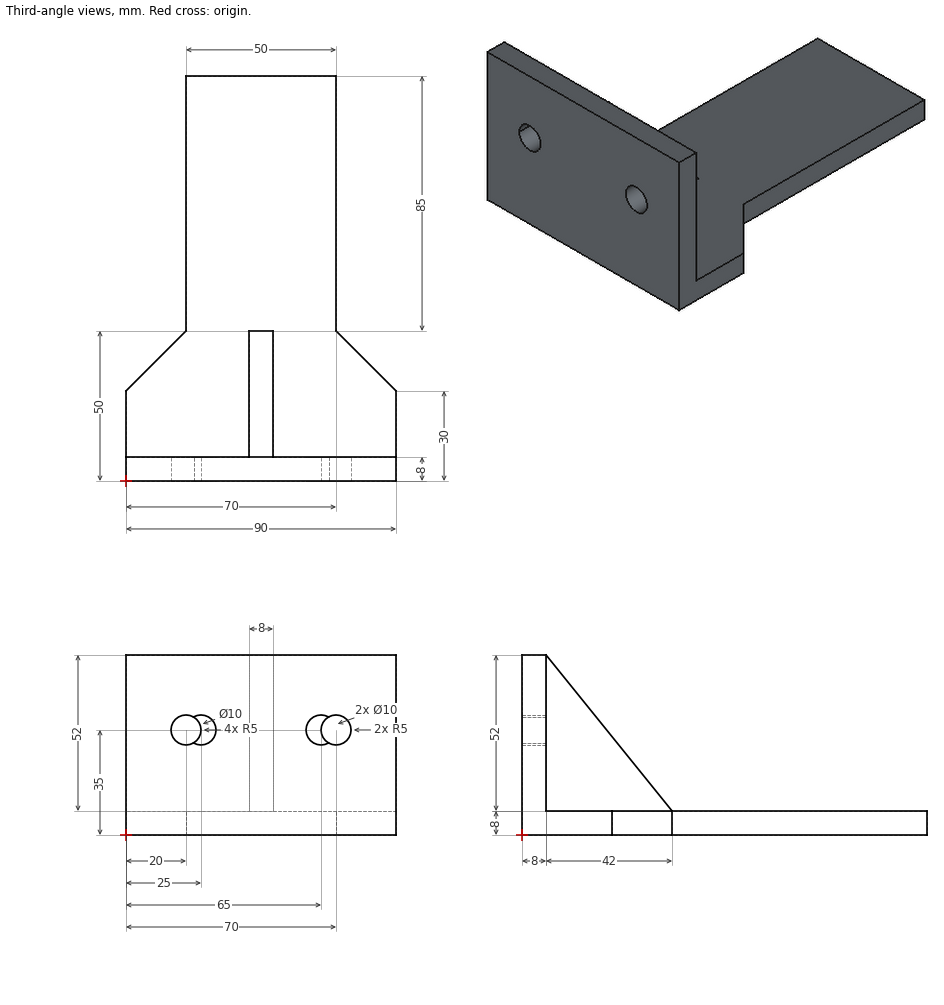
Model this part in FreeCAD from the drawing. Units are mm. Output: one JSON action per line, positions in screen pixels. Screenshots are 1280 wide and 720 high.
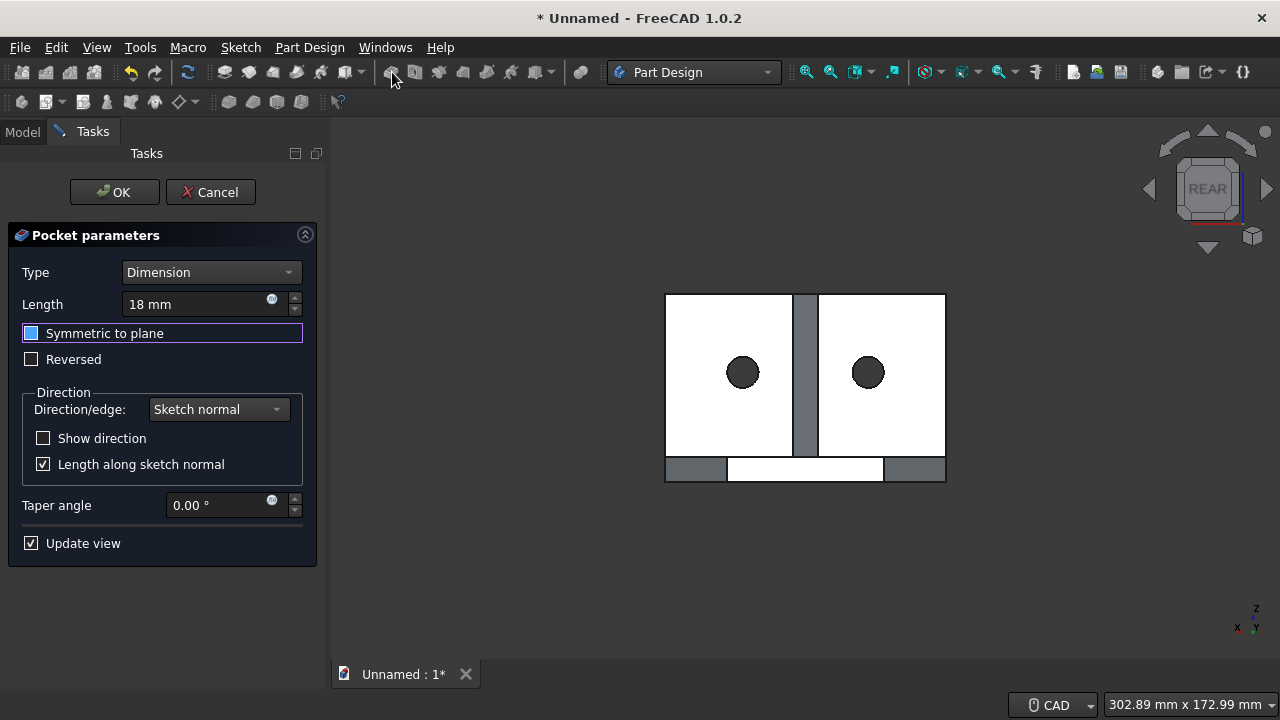
{"action": "left_click", "coordinate": [115, 192]}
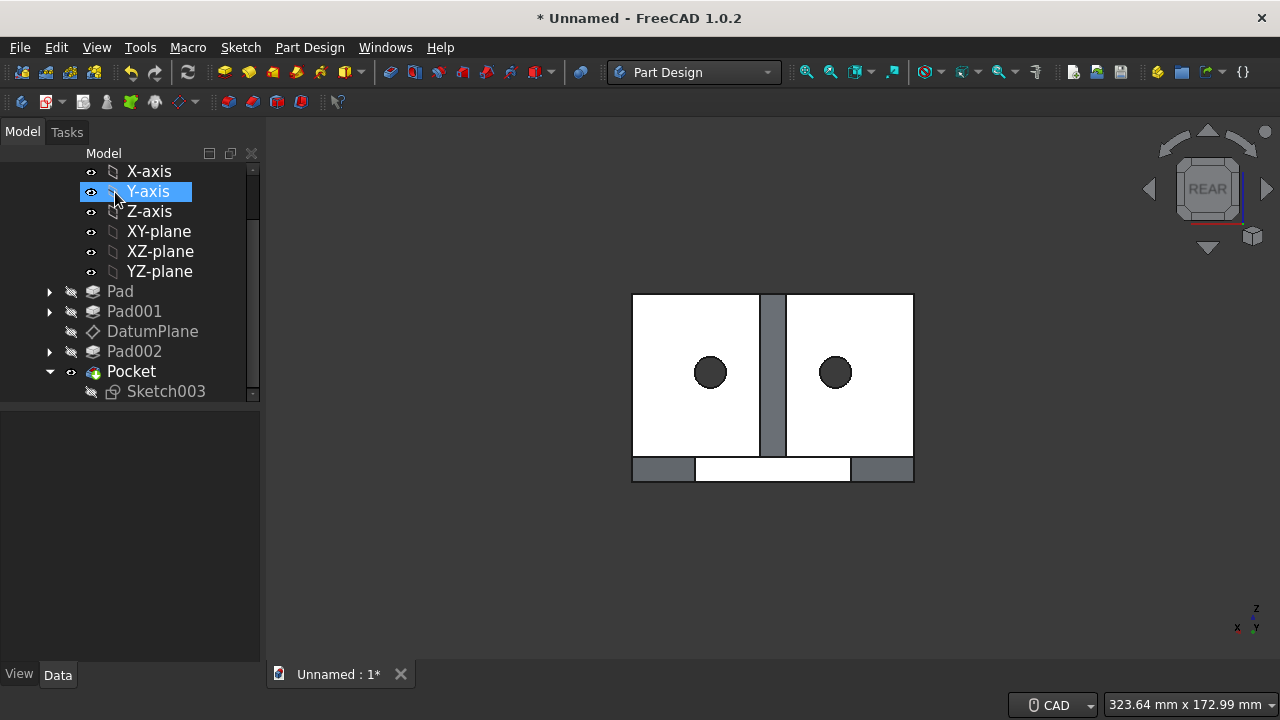
{"action": "left_click", "coordinate": [808, 72]}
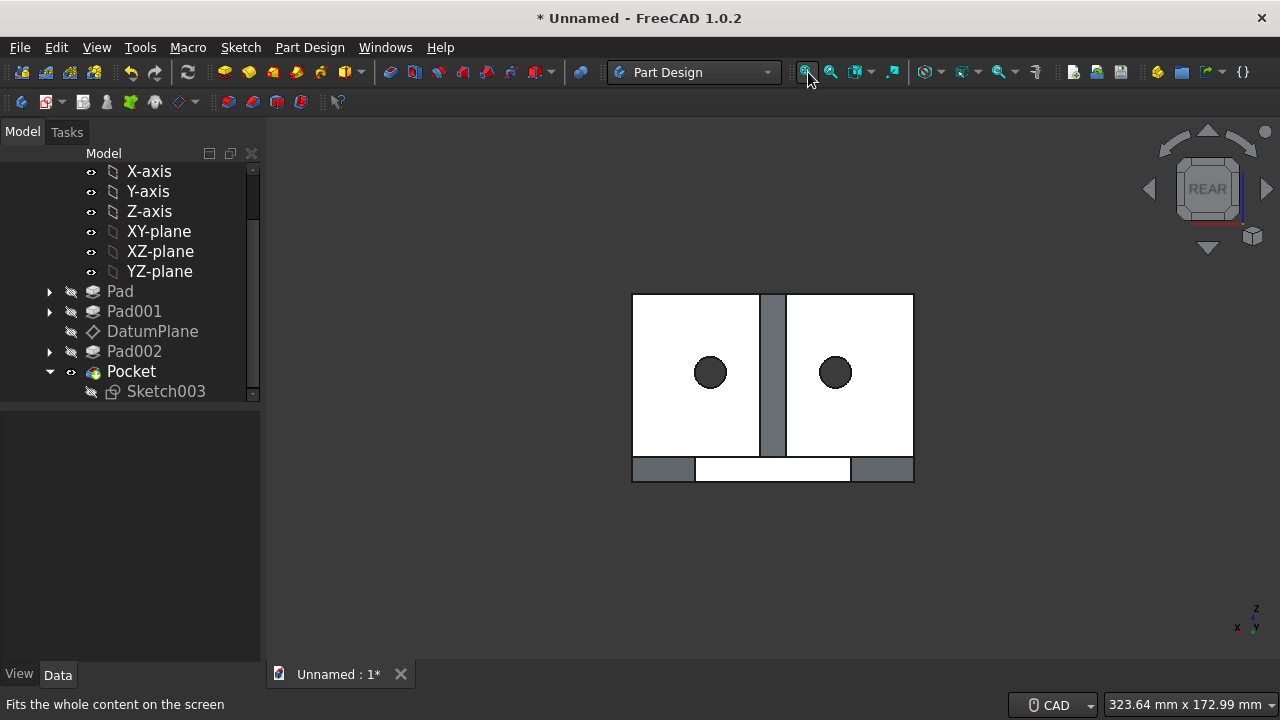
{"action": "left_click", "coordinate": [850, 421]}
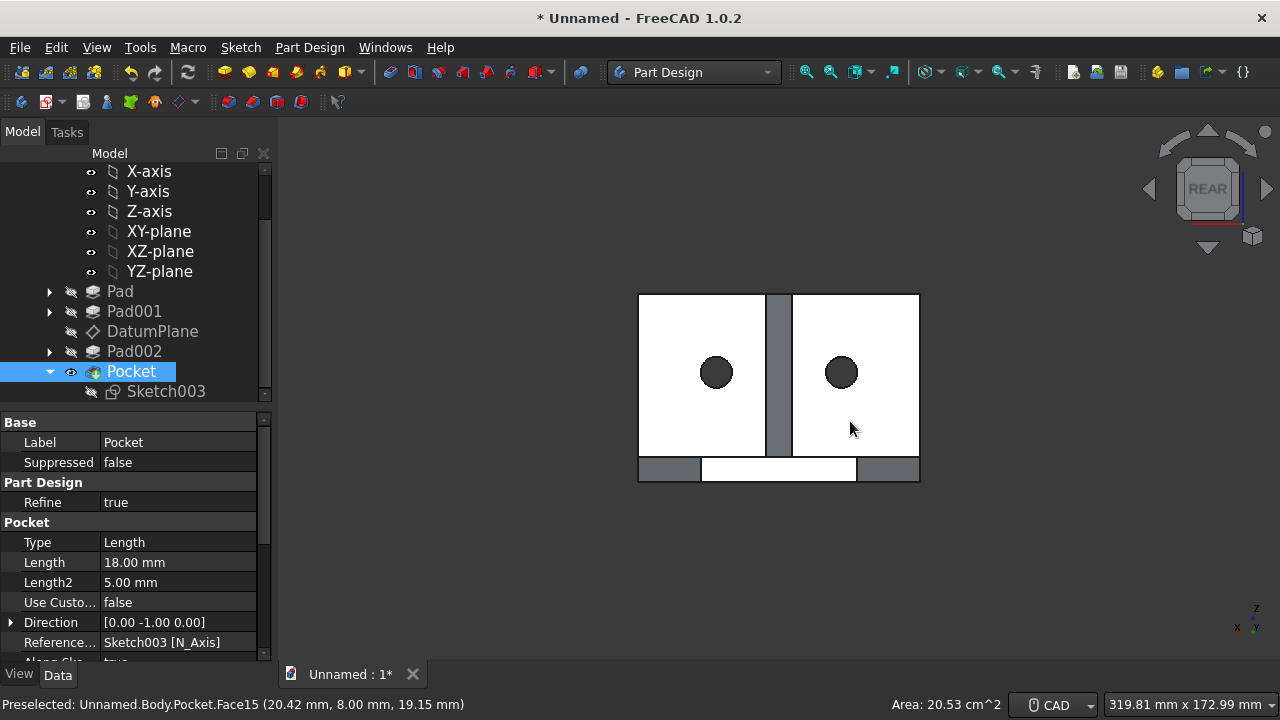
{"action": "left_click", "coordinate": [46, 102]}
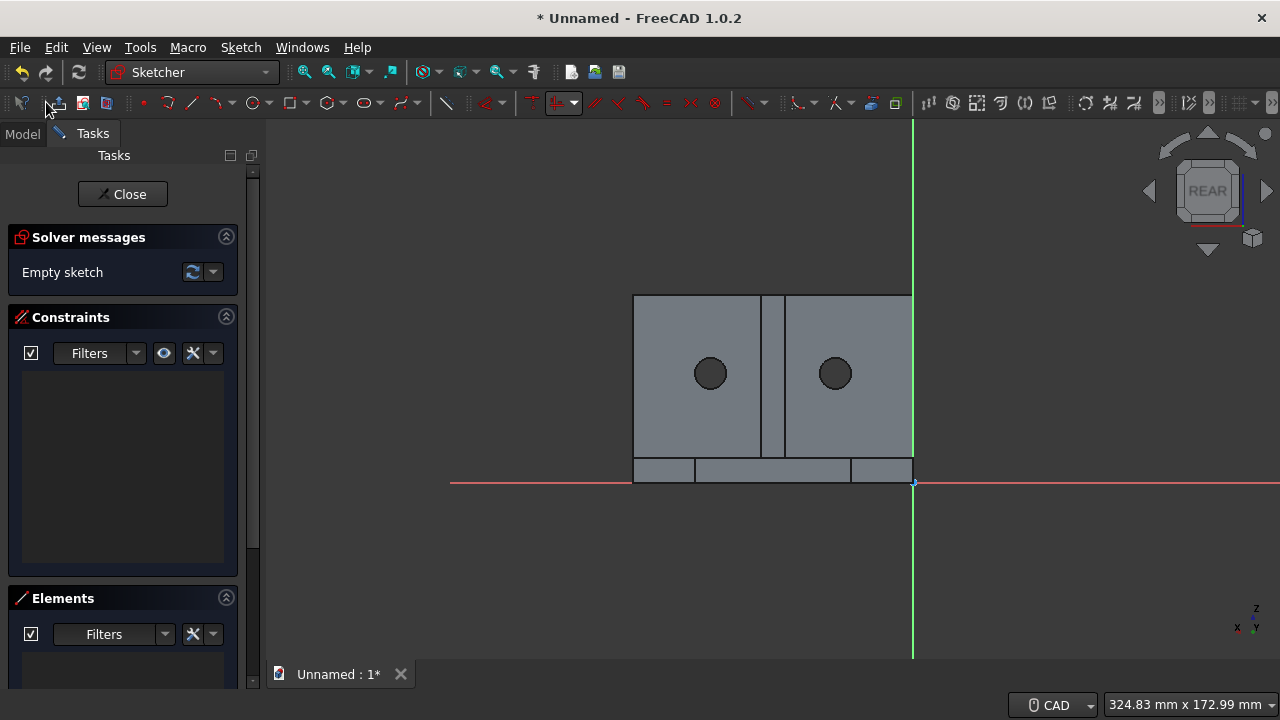
{"action": "left_click", "coordinate": [108, 104]}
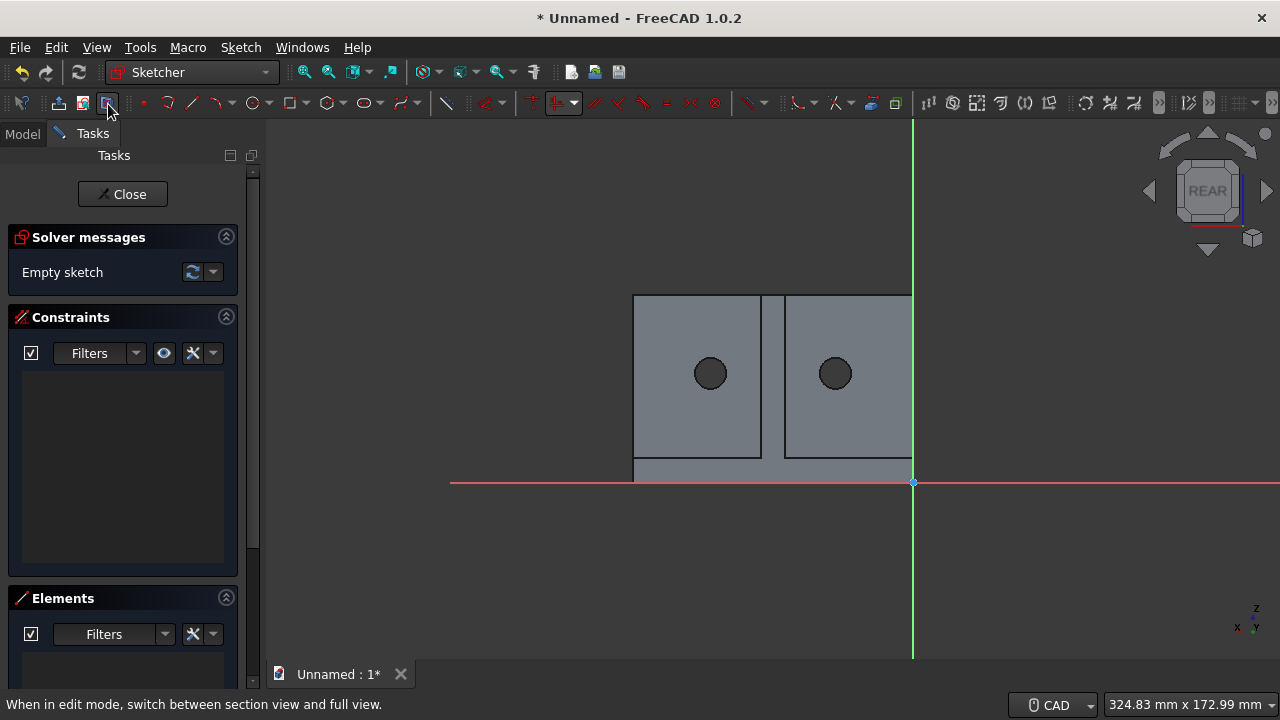
{"action": "scroll", "coordinate": [866, 372], "scroll_direction": "up", "scroll_amount": 12}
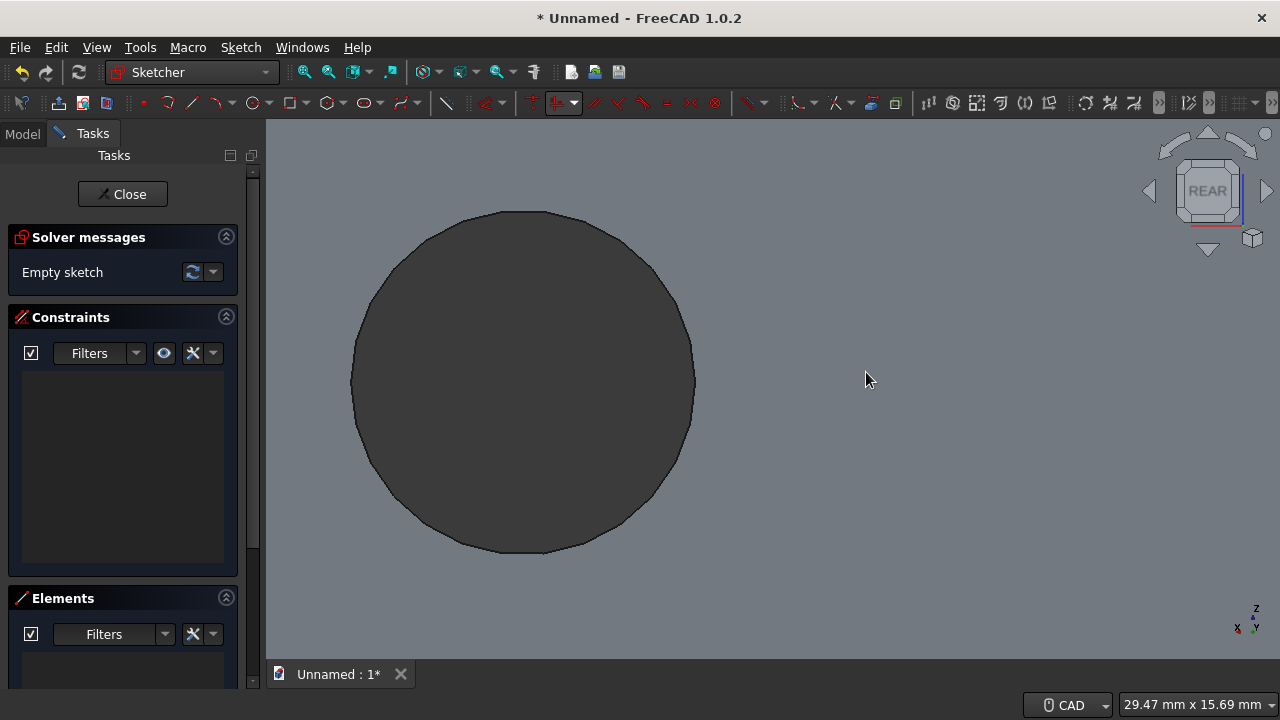
{"action": "left_click", "coordinate": [254, 104]}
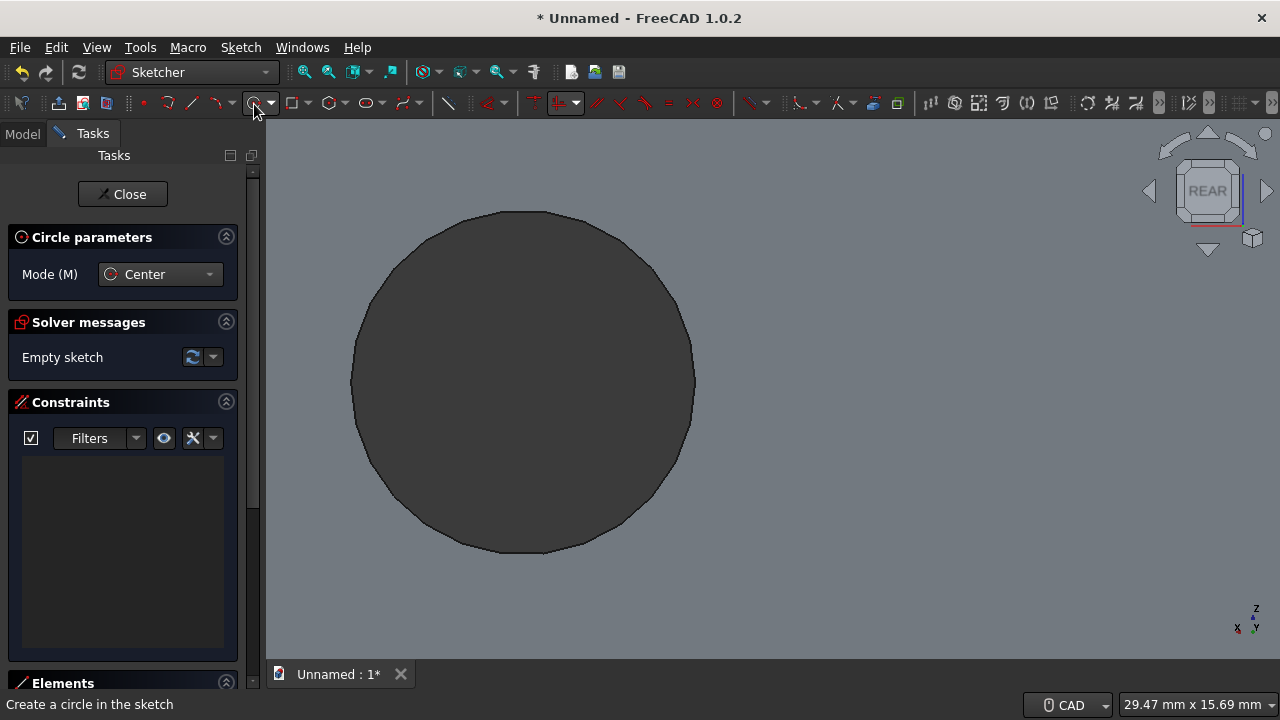
{"action": "left_click", "coordinate": [695, 383]}
{"action": "mouse_move", "coordinate": [817, 261]}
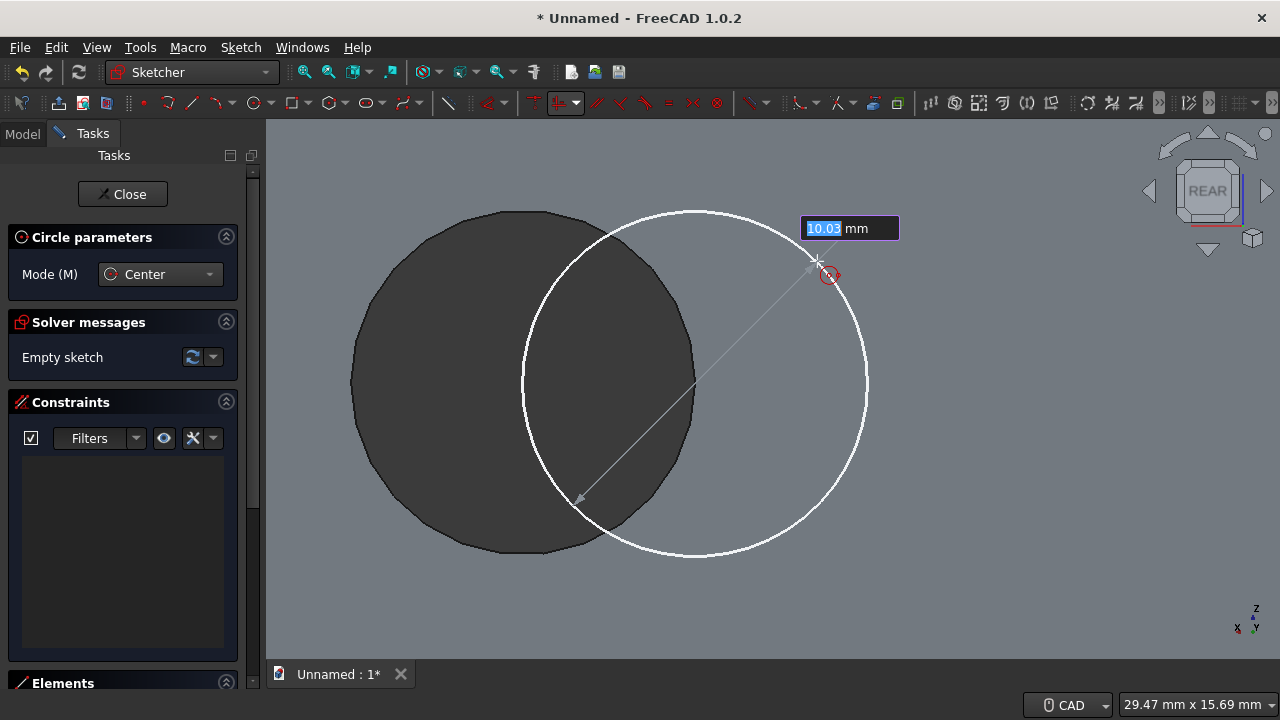
{"action": "type", "text": "10"}
{"action": "key", "text": "Return"}
{"action": "key", "text": "Escape"}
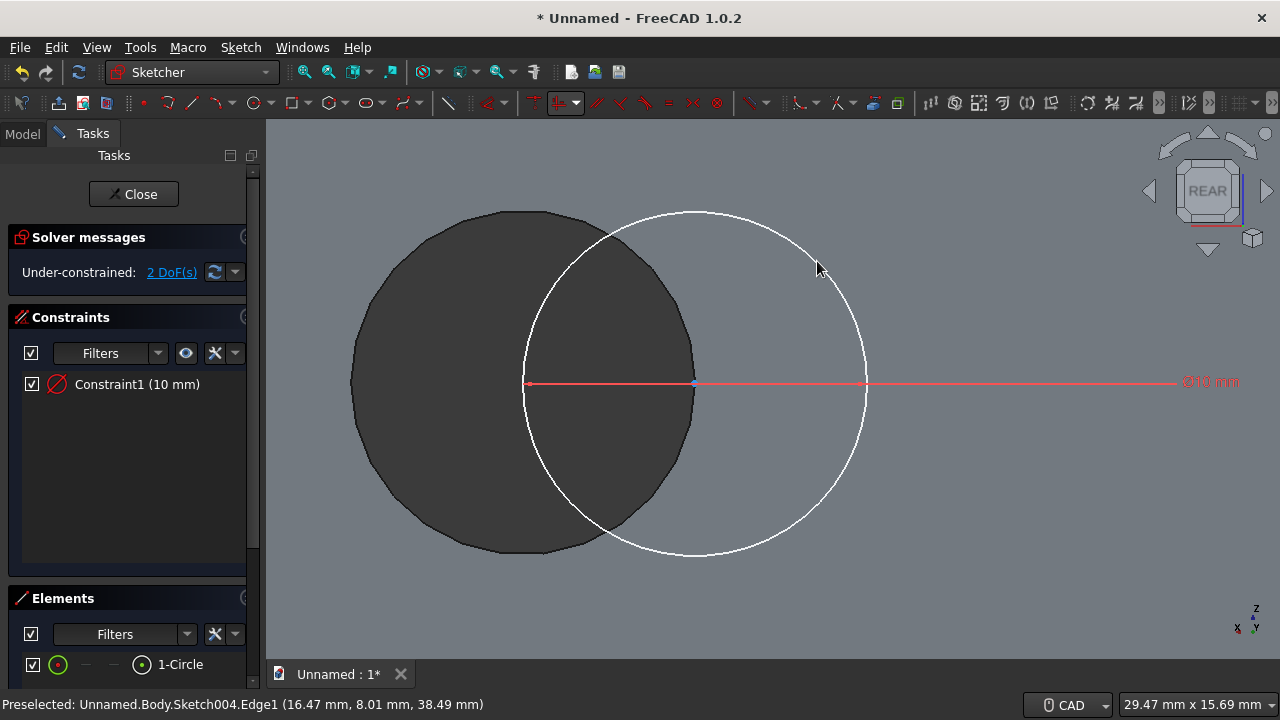
{"action": "left_click", "coordinate": [488, 104]}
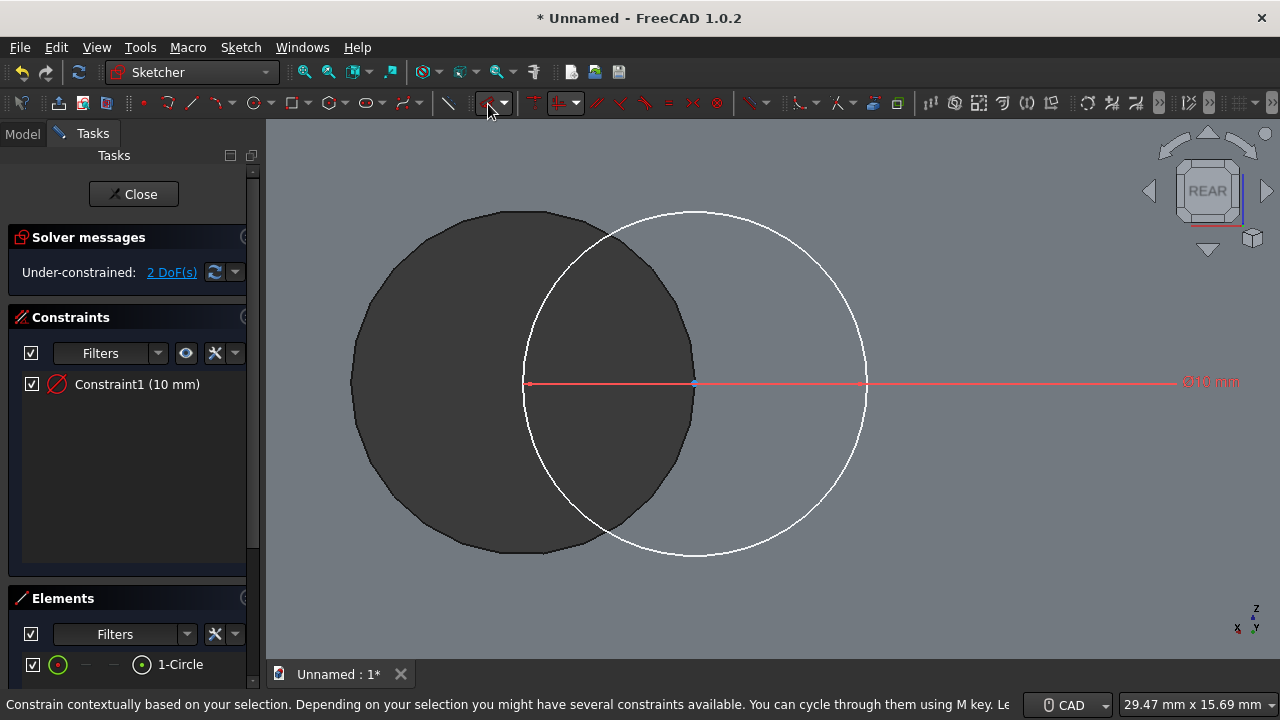
{"action": "left_click", "coordinate": [695, 384]}
{"action": "left_click", "coordinate": [905, 350]}